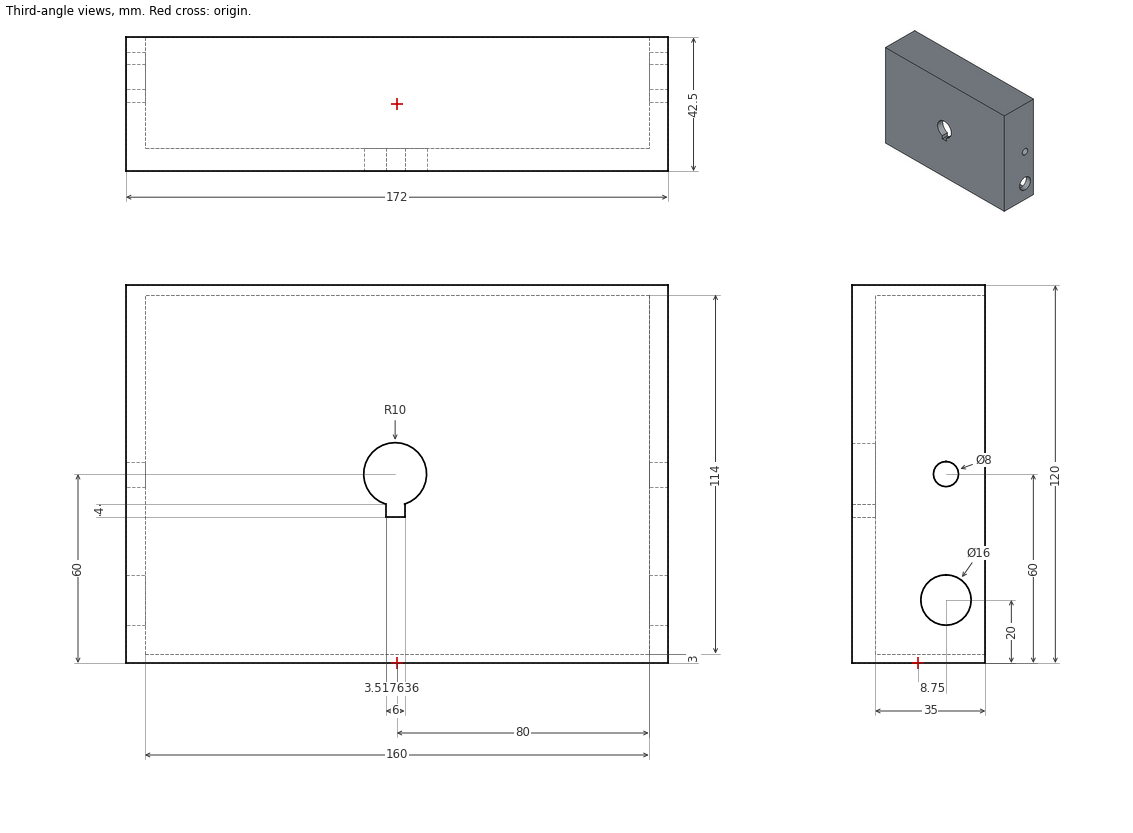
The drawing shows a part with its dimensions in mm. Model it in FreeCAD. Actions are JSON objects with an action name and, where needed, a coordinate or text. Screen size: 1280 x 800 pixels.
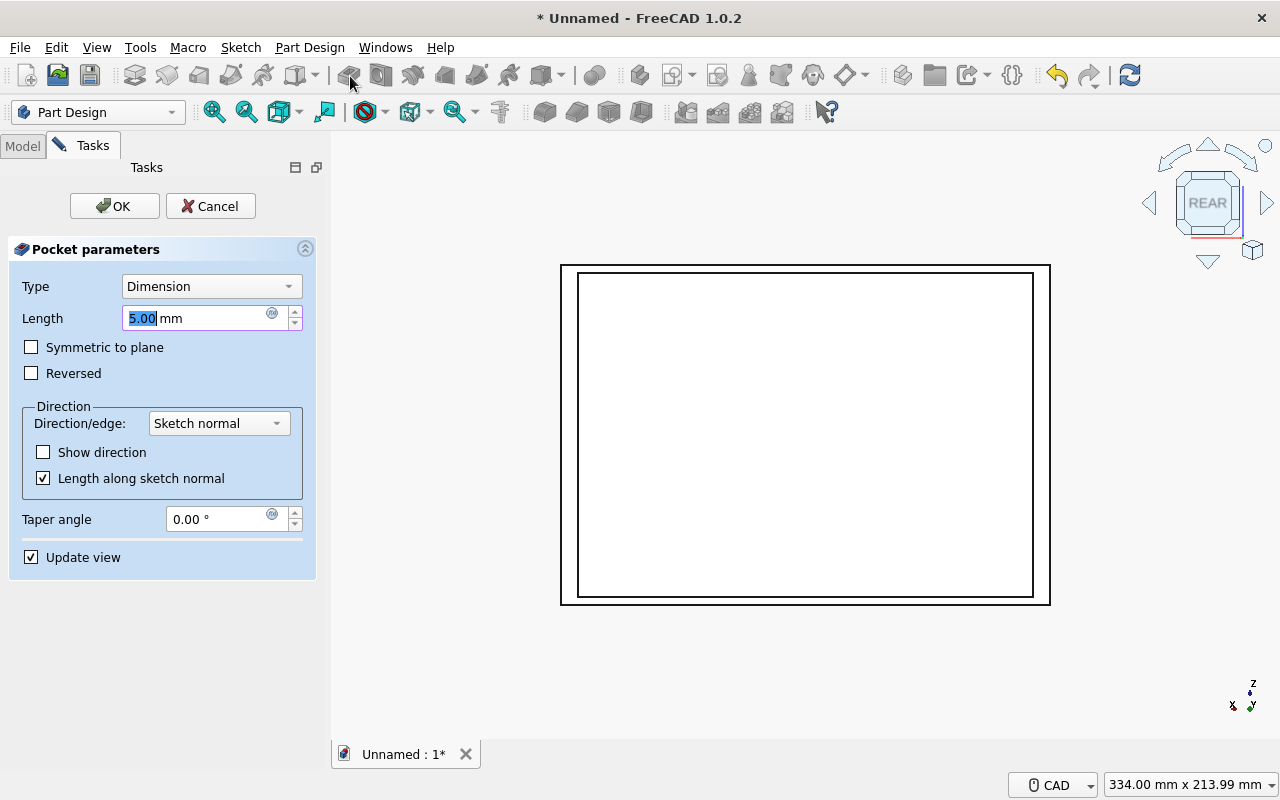
{"action": "type", "text": "35"}
{"action": "key", "text": "Tab"}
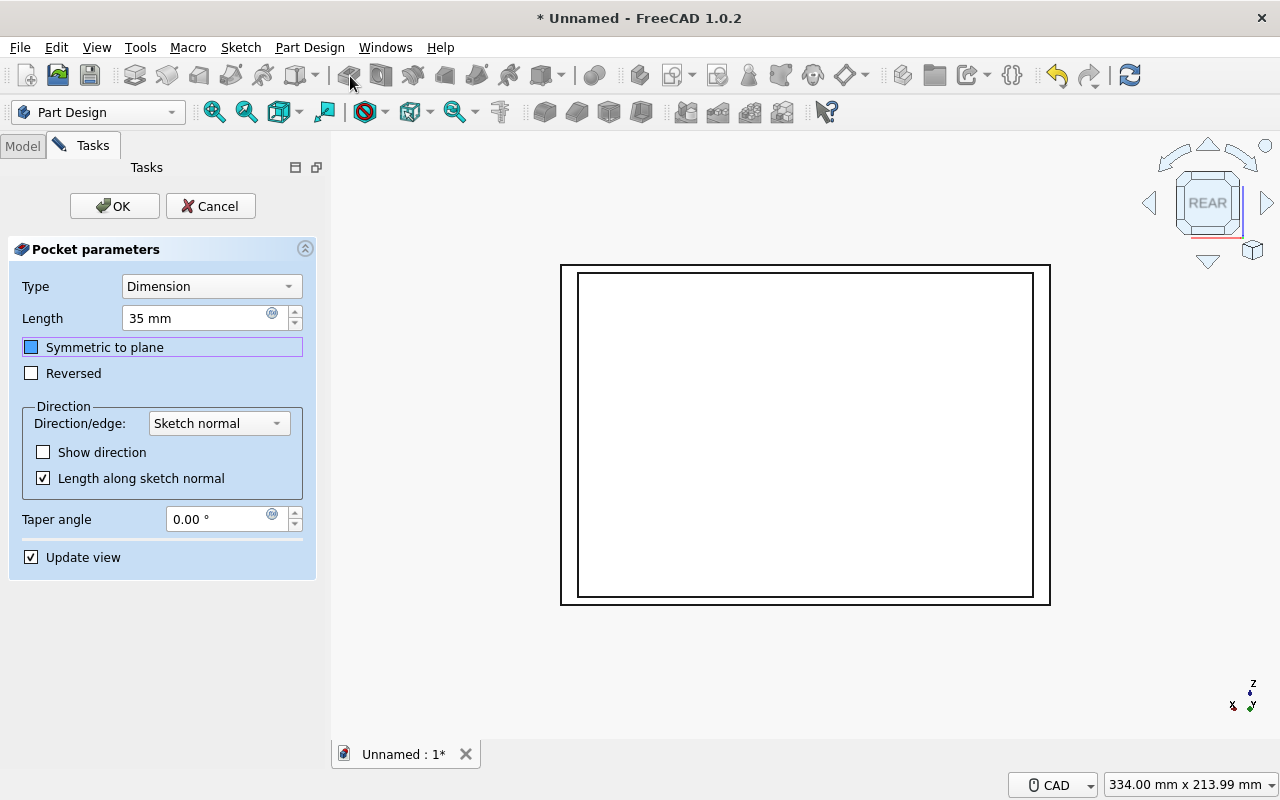
{"action": "left_click", "coordinate": [115, 206]}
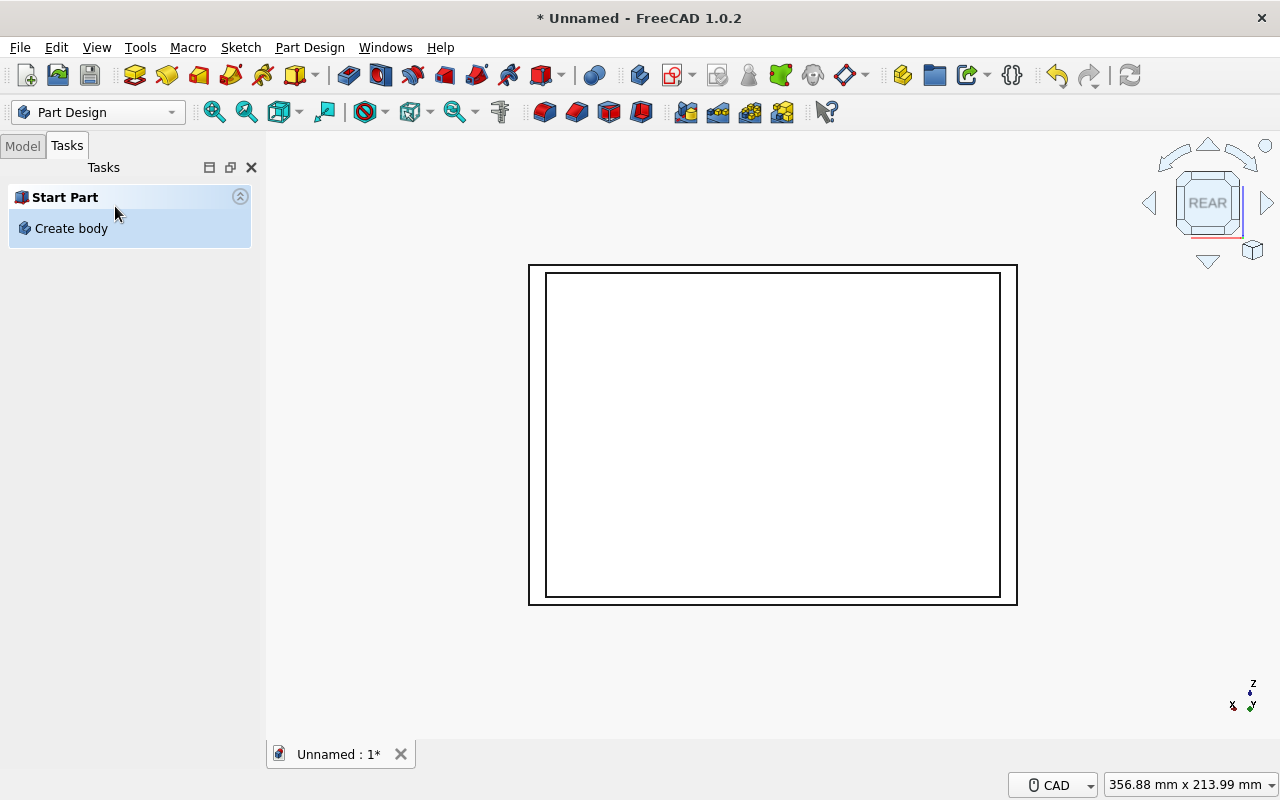
{"action": "key", "text": "6"}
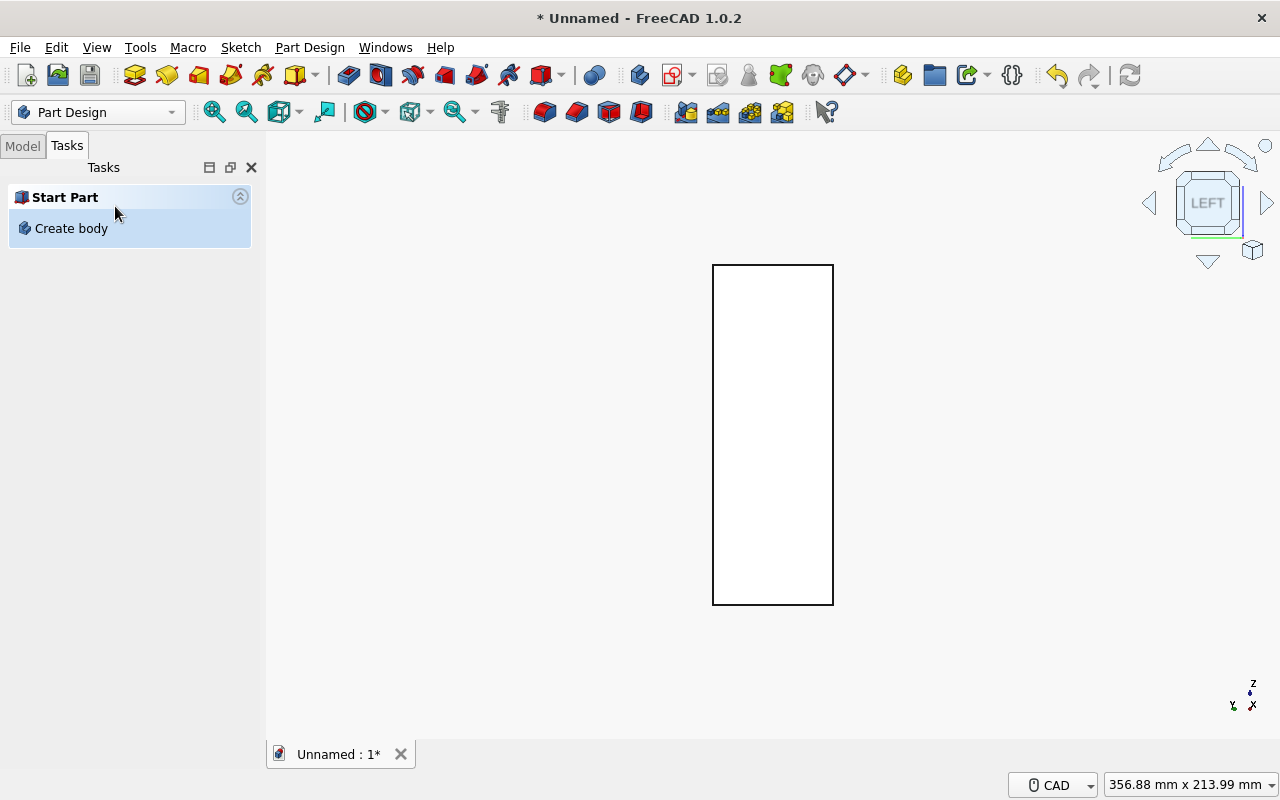
{"action": "left_click", "coordinate": [773, 337]}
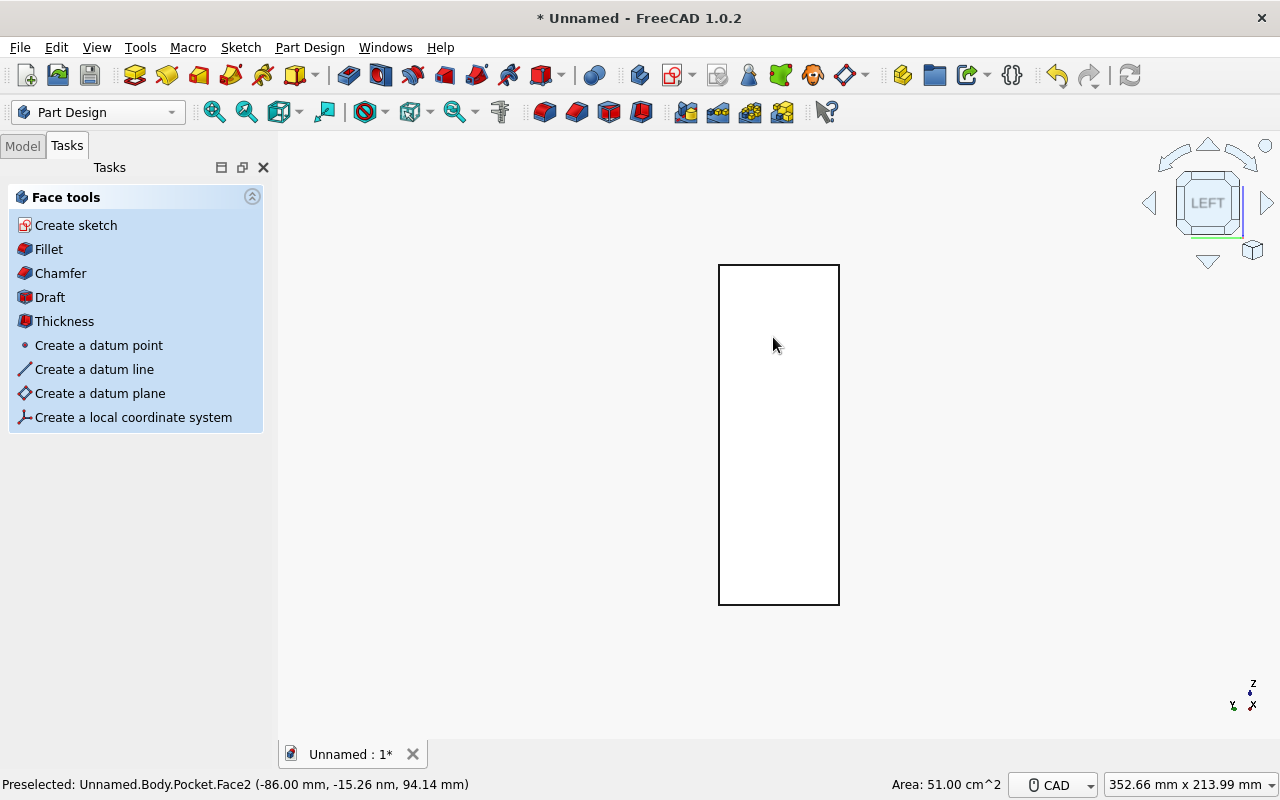
{"action": "left_click", "coordinate": [672, 76]}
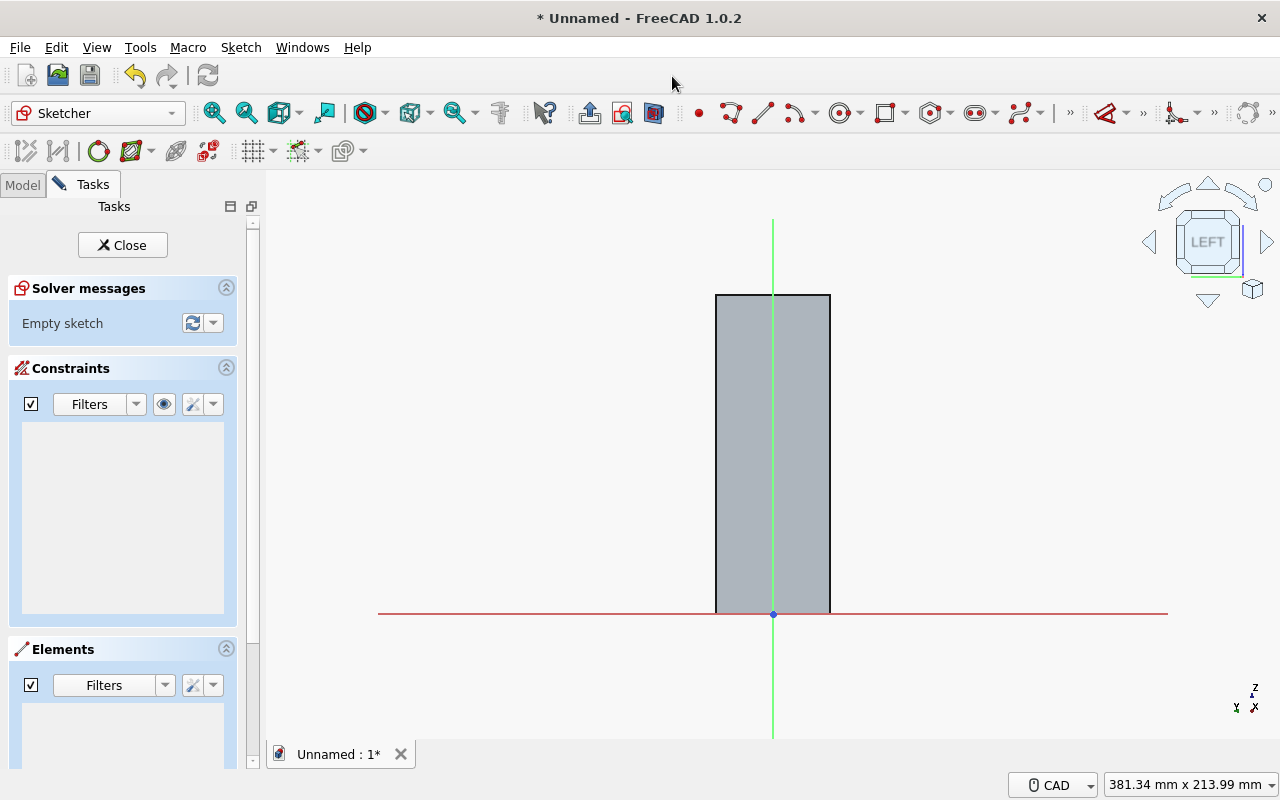
{"action": "scroll", "coordinate": [788, 590], "scroll_direction": "up", "scroll_amount": 4}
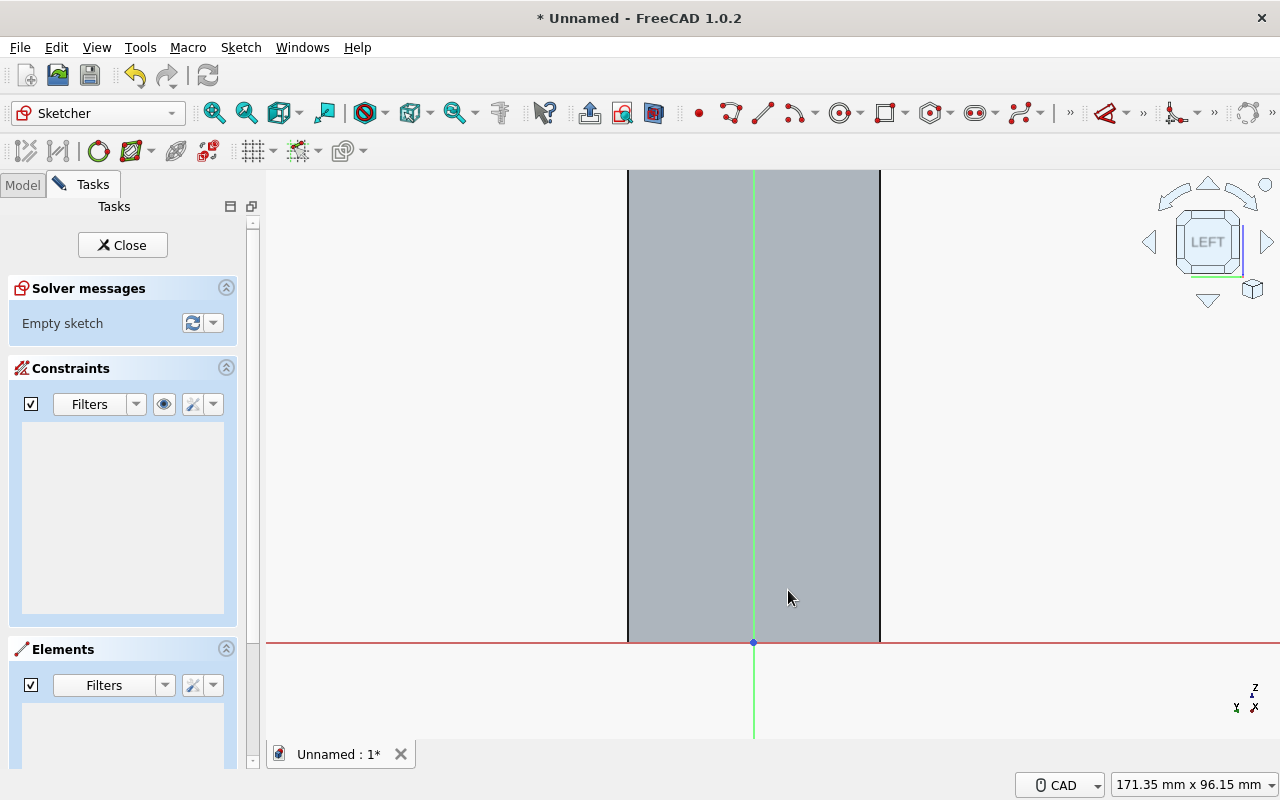
{"action": "left_click", "coordinate": [840, 114]}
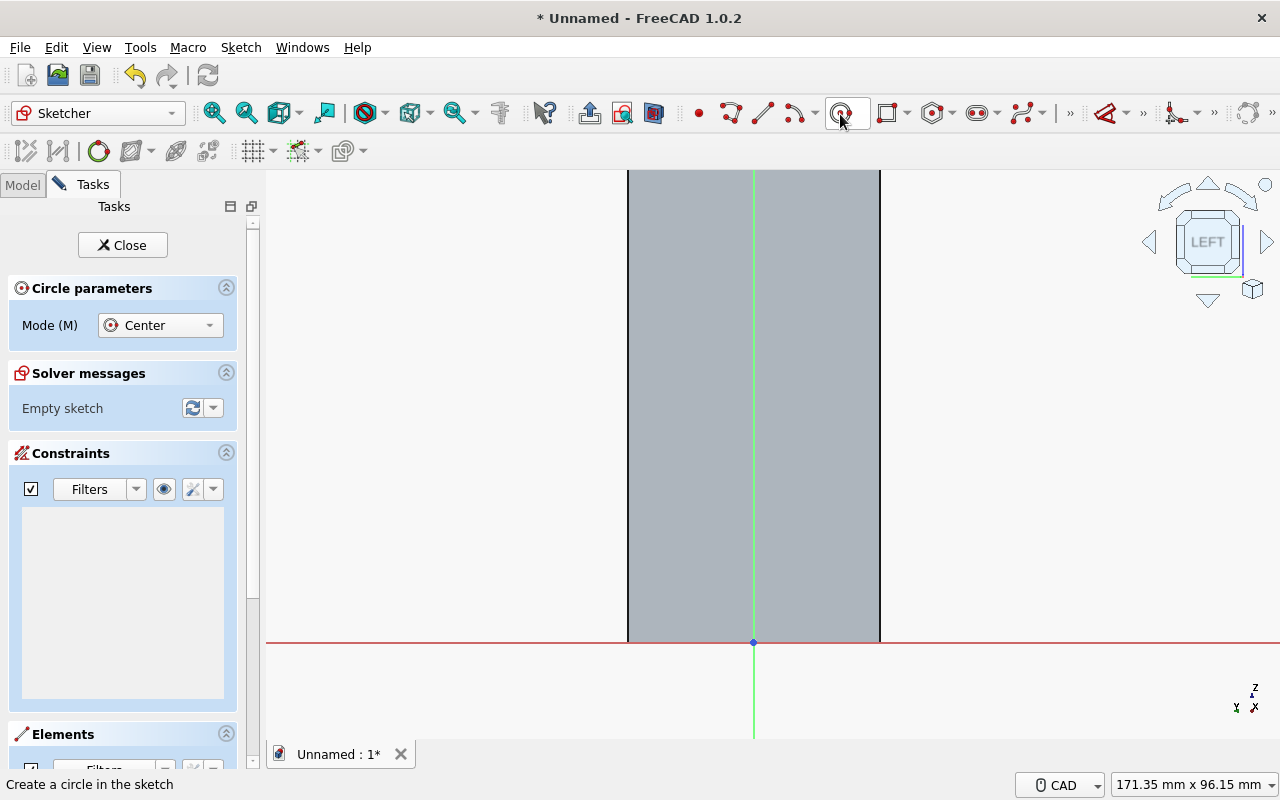
{"action": "left_click", "coordinate": [702, 524]}
{"action": "left_click", "coordinate": [736, 491]}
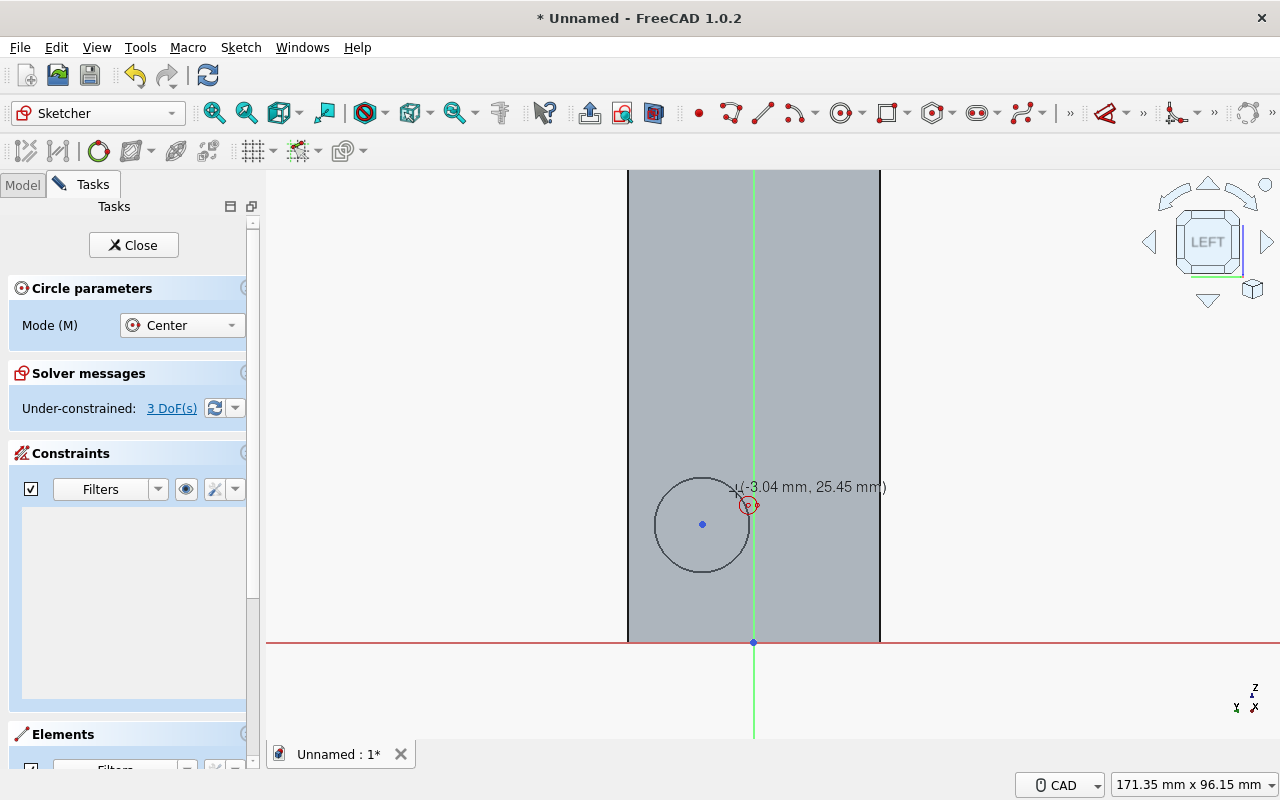
{"action": "left_click", "coordinate": [702, 288]}
{"action": "left_click", "coordinate": [719, 271]}
{"action": "key", "text": "Escape"}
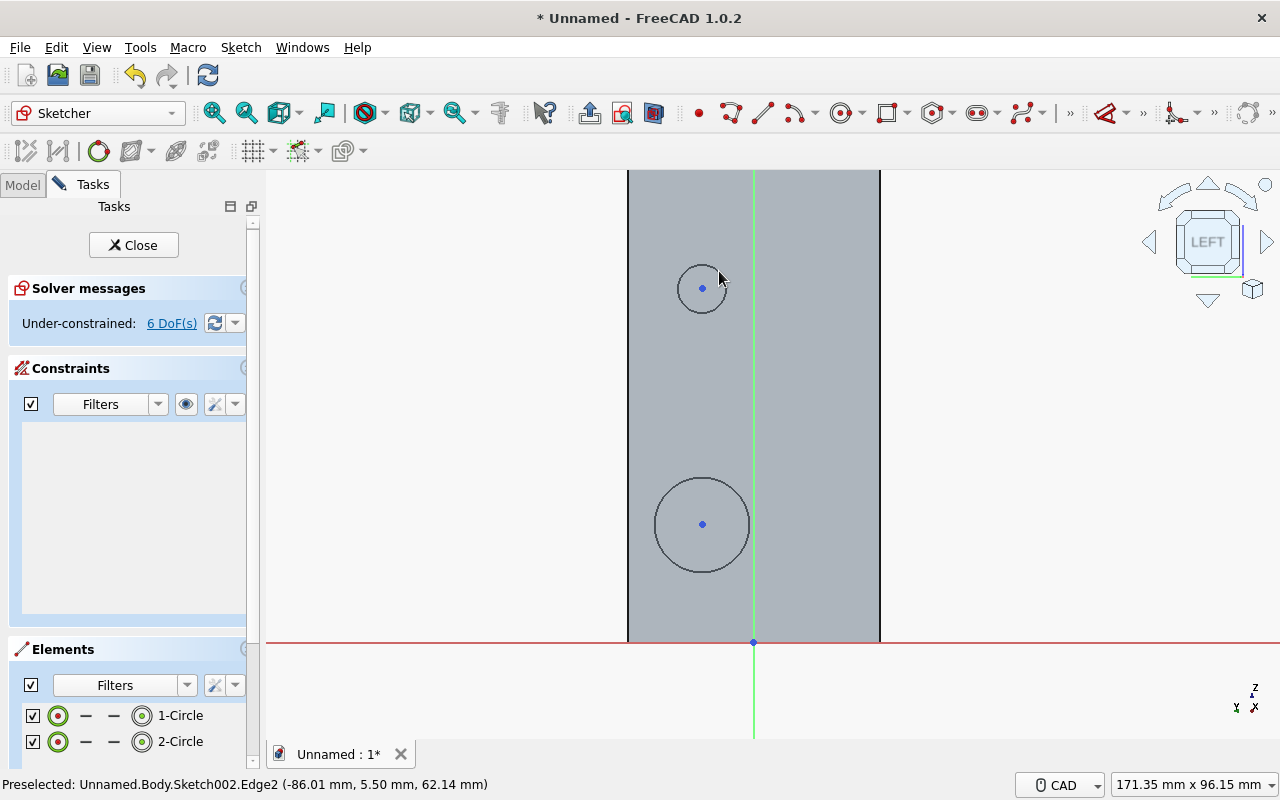
{"action": "left_click", "coordinate": [702, 525]}